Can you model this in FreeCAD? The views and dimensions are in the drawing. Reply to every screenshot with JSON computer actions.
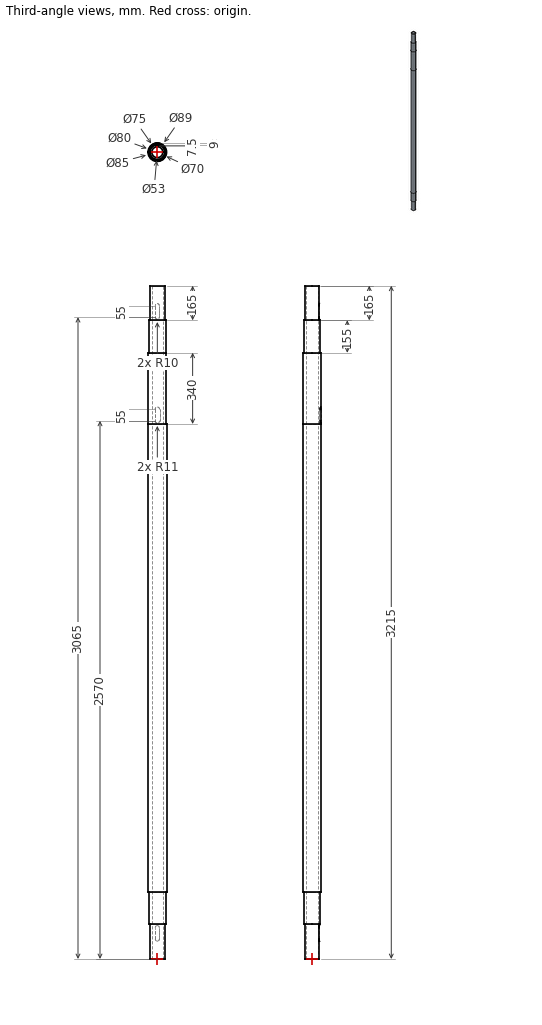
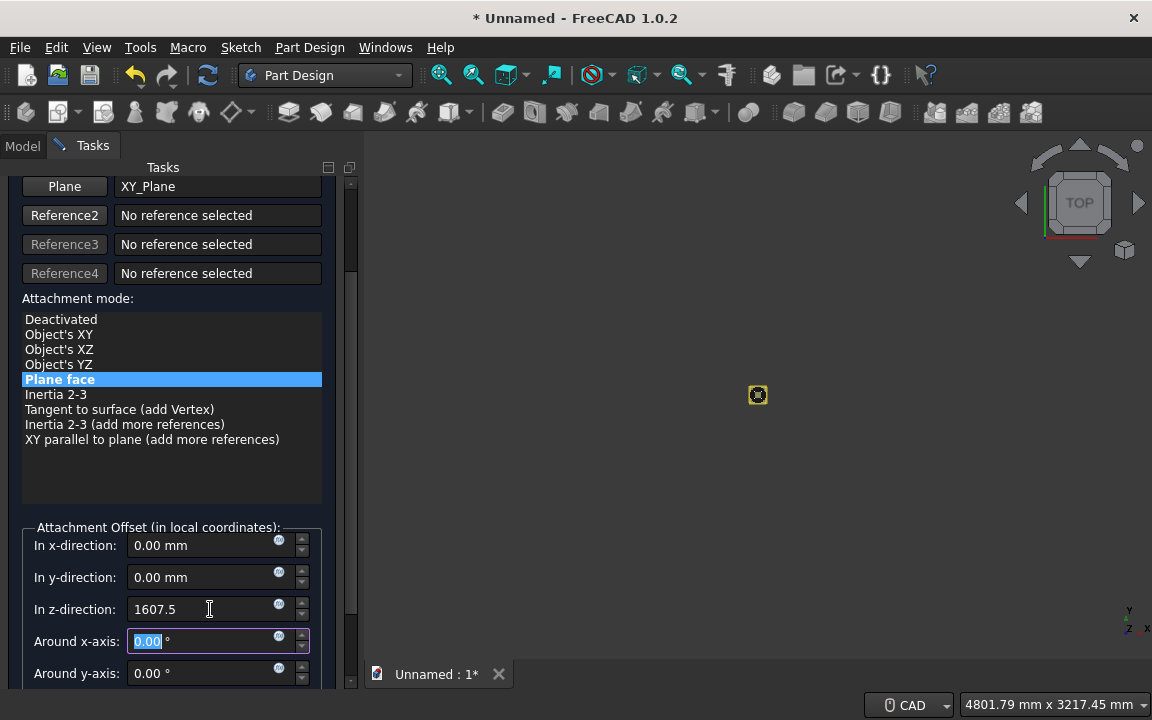
{"action": "scroll", "coordinate": [351, 432], "scroll_direction": "up", "scroll_amount": 3}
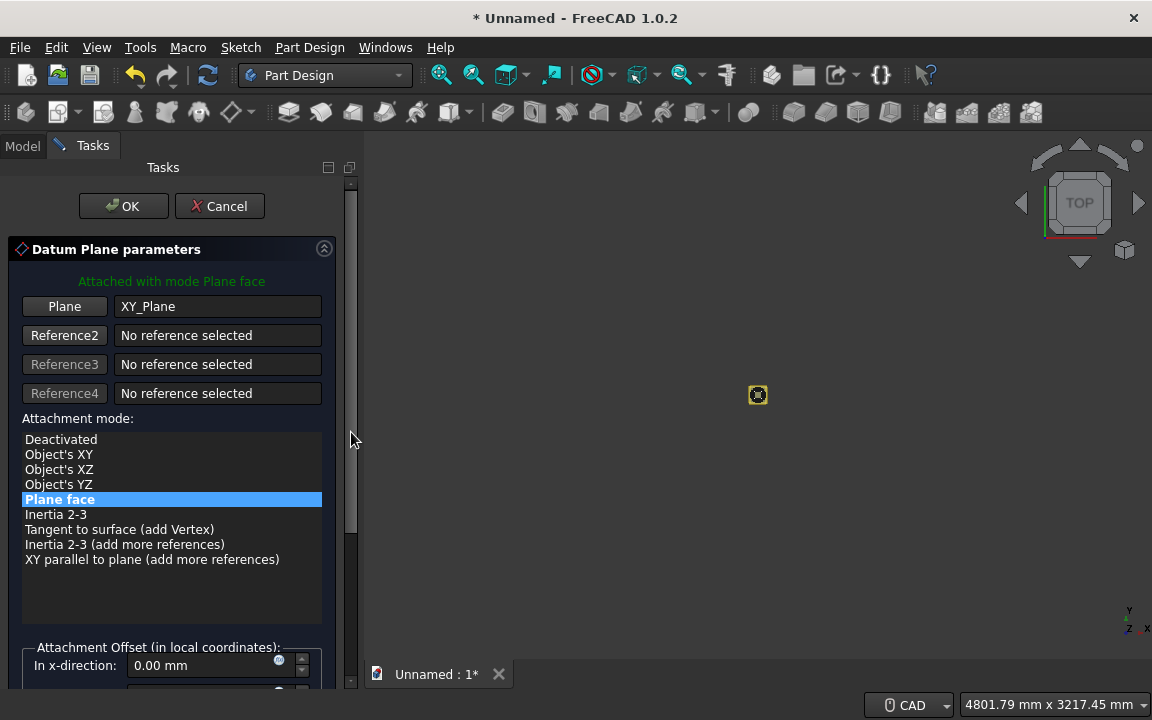
{"action": "left_click", "coordinate": [124, 206]}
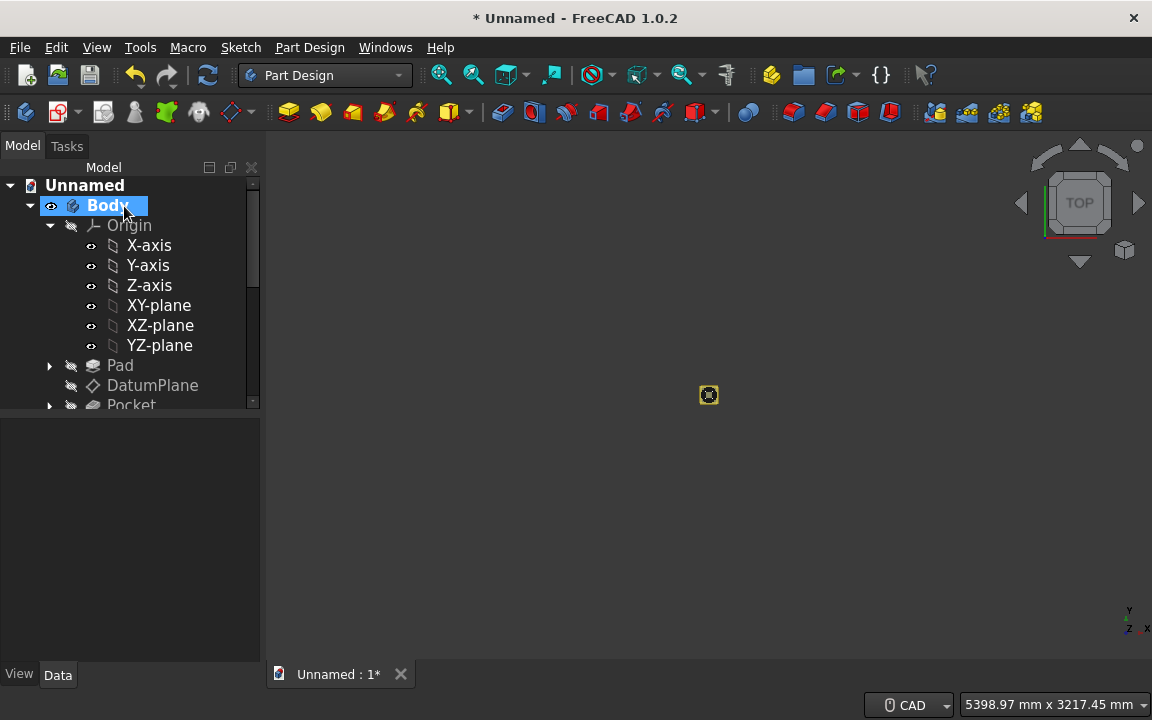
{"action": "scroll", "coordinate": [100, 301], "scroll_direction": "down", "scroll_amount": 3}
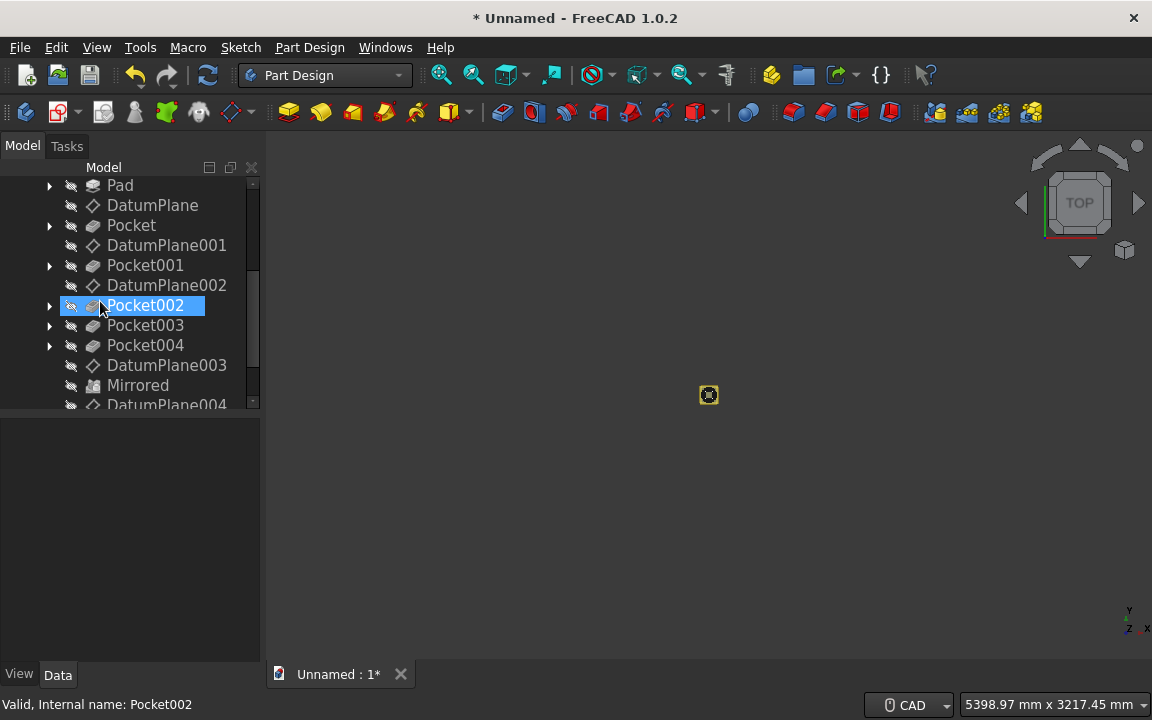
{"action": "scroll", "coordinate": [140, 301], "scroll_direction": "up", "scroll_amount": 15}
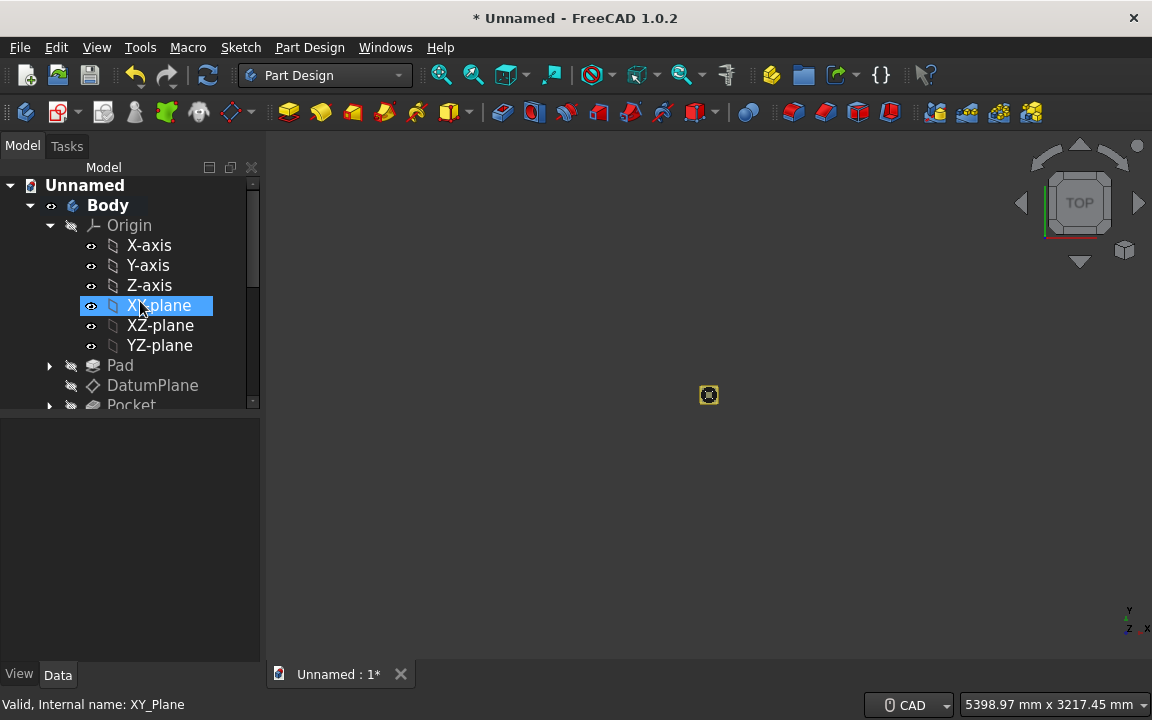
{"action": "scroll", "coordinate": [100, 301], "scroll_direction": "down", "scroll_amount": 6}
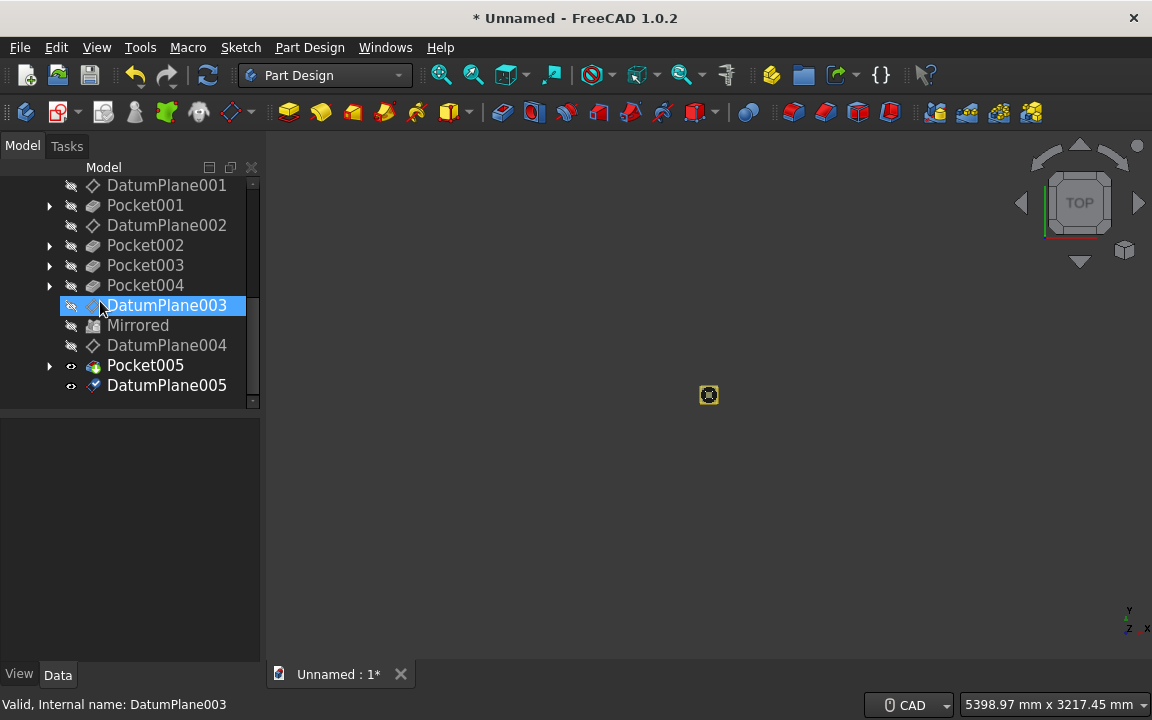
{"action": "left_click", "coordinate": [116, 366]}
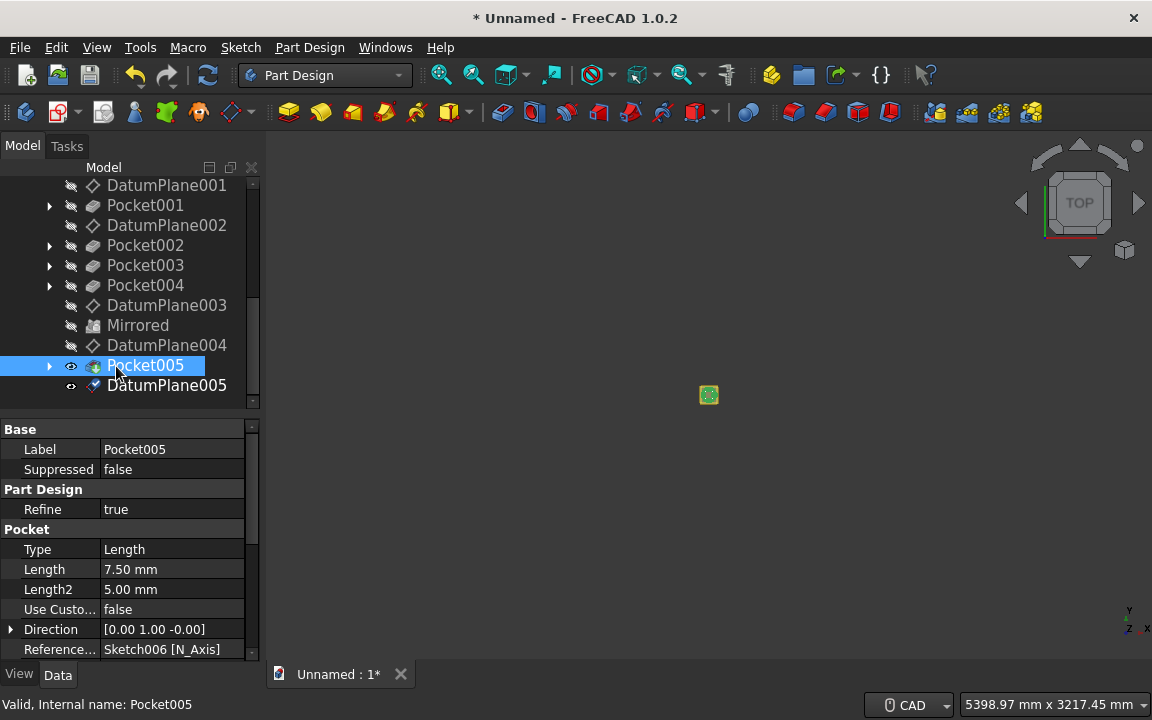
{"action": "left_click", "coordinate": [936, 112]}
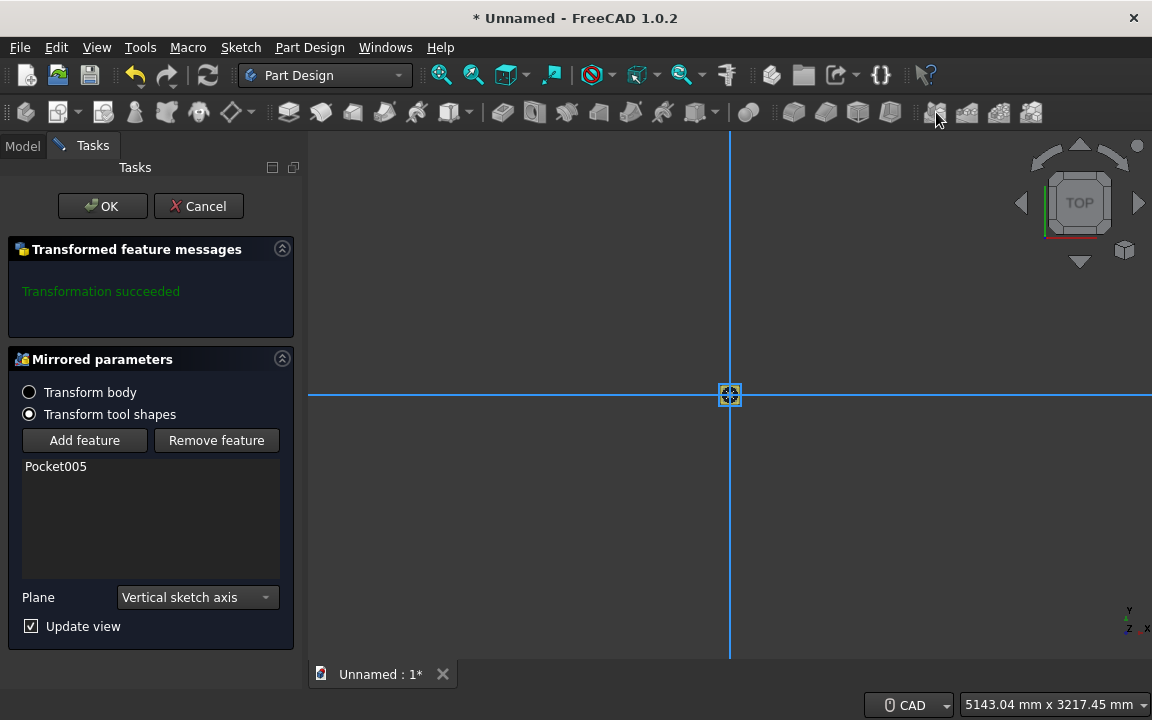
{"action": "left_click", "coordinate": [198, 598]}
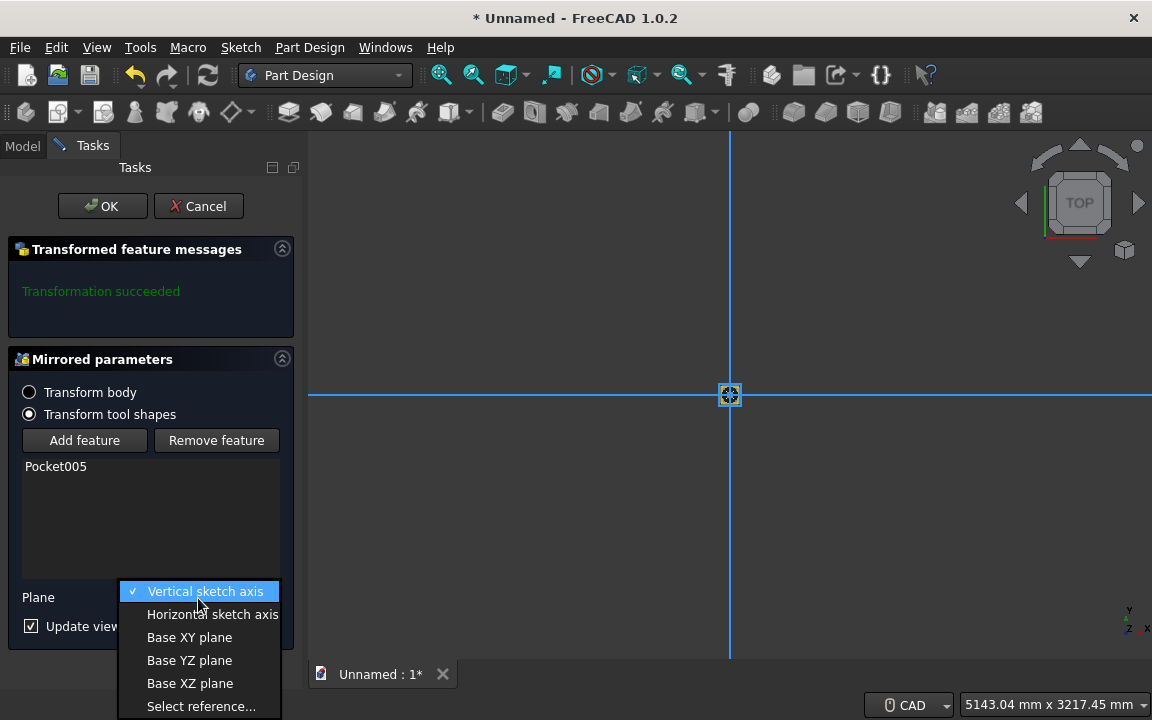
{"action": "left_click", "coordinate": [198, 706]}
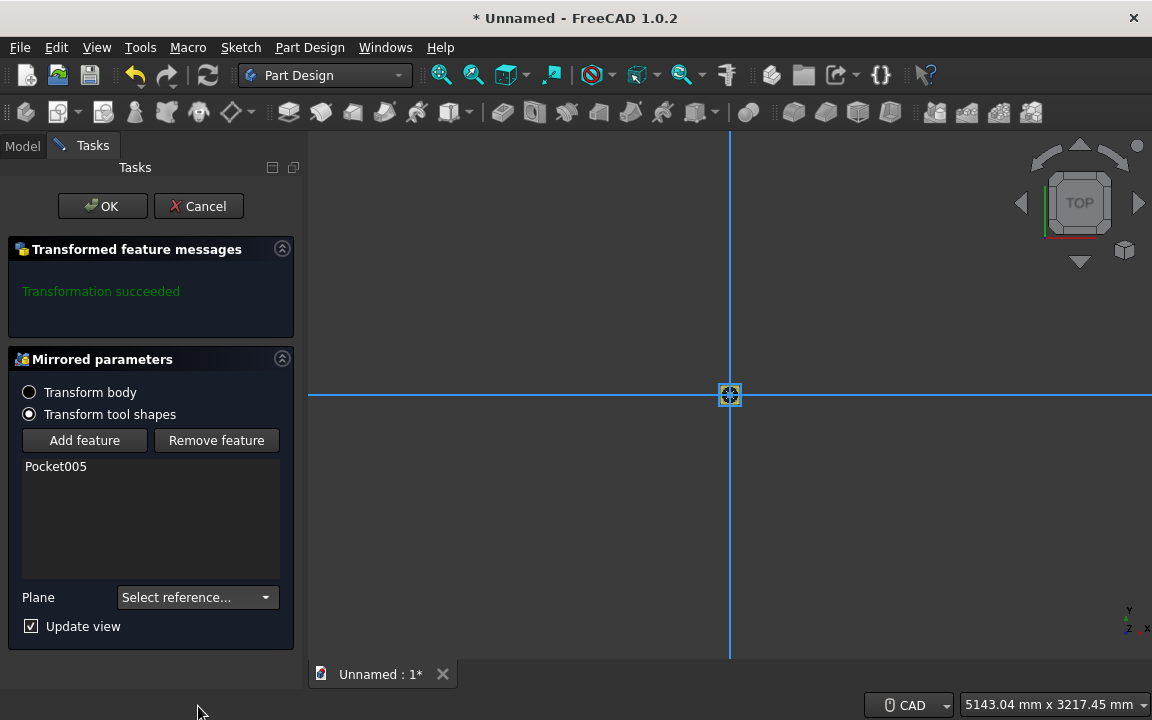
{"action": "left_click", "coordinate": [23, 145]}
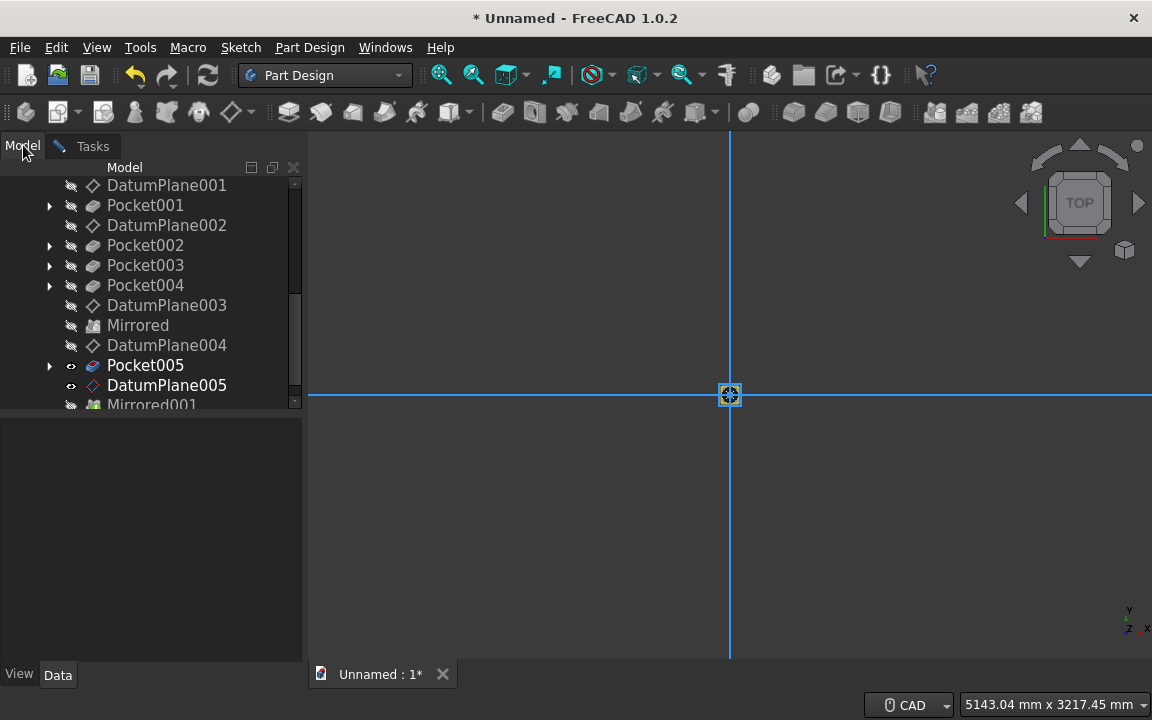
{"action": "left_click", "coordinate": [116, 386]}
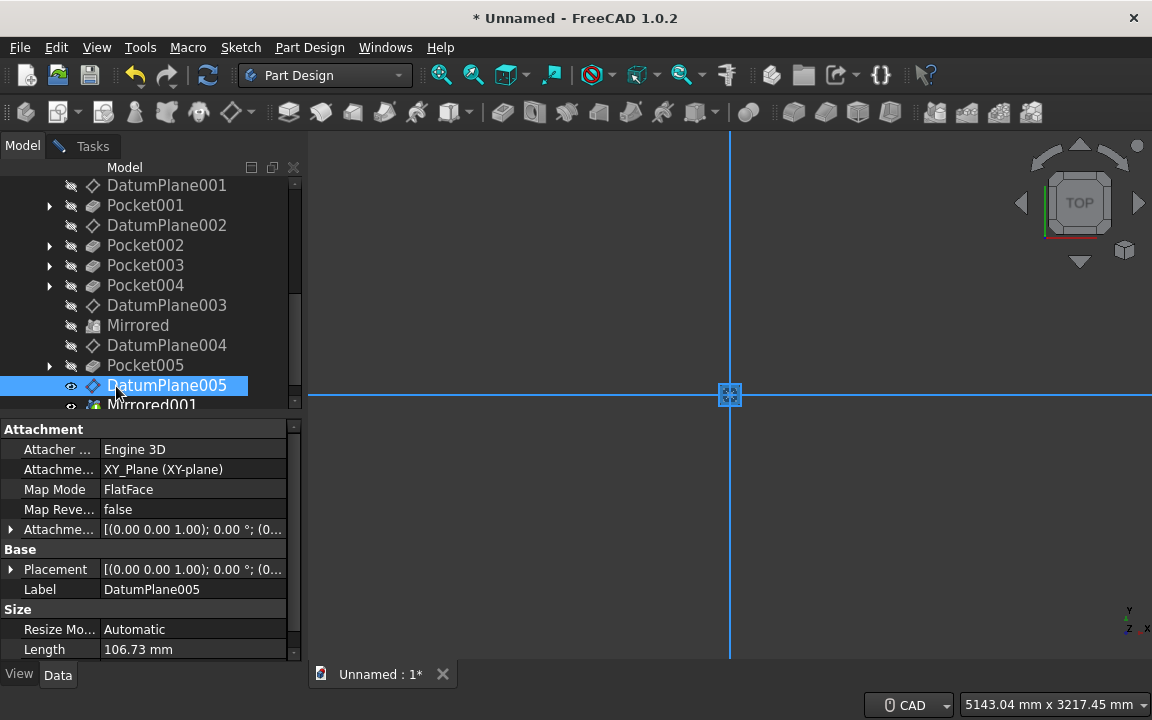
{"action": "left_click", "coordinate": [84, 145]}